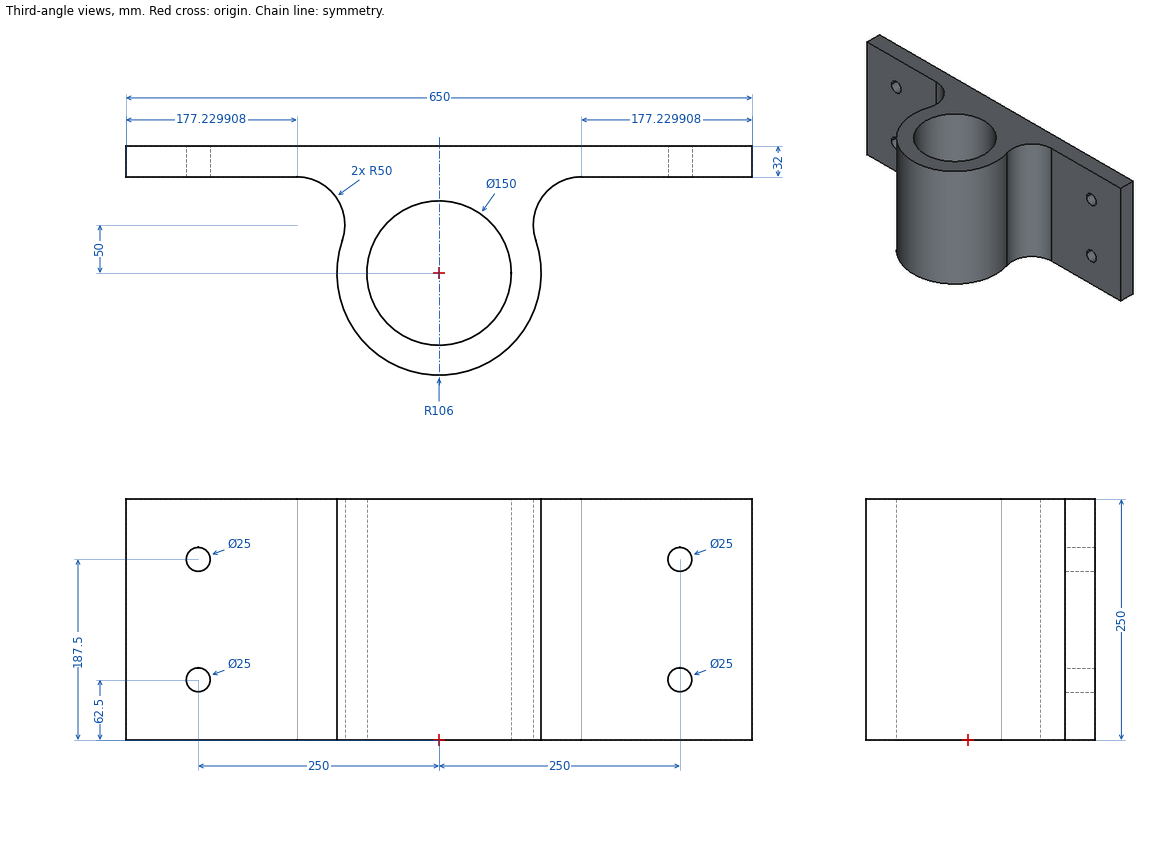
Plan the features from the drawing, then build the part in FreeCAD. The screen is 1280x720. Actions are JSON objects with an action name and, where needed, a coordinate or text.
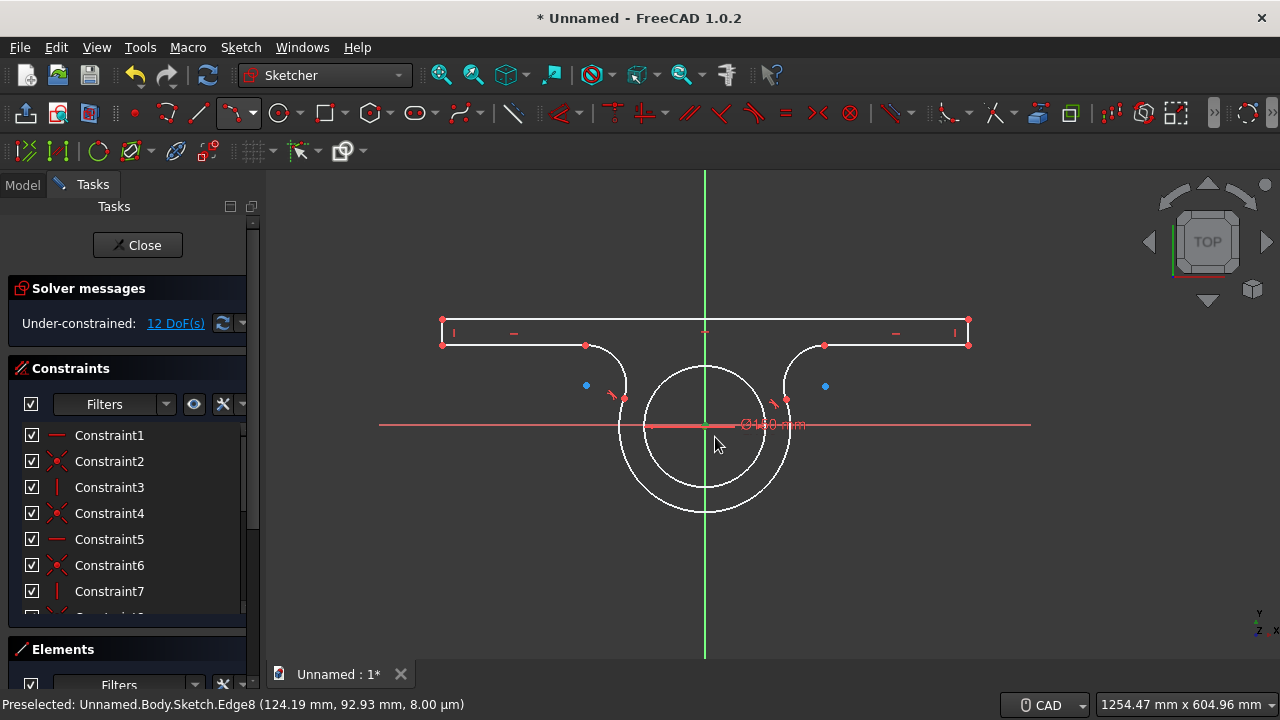
{"action": "key", "text": "c"}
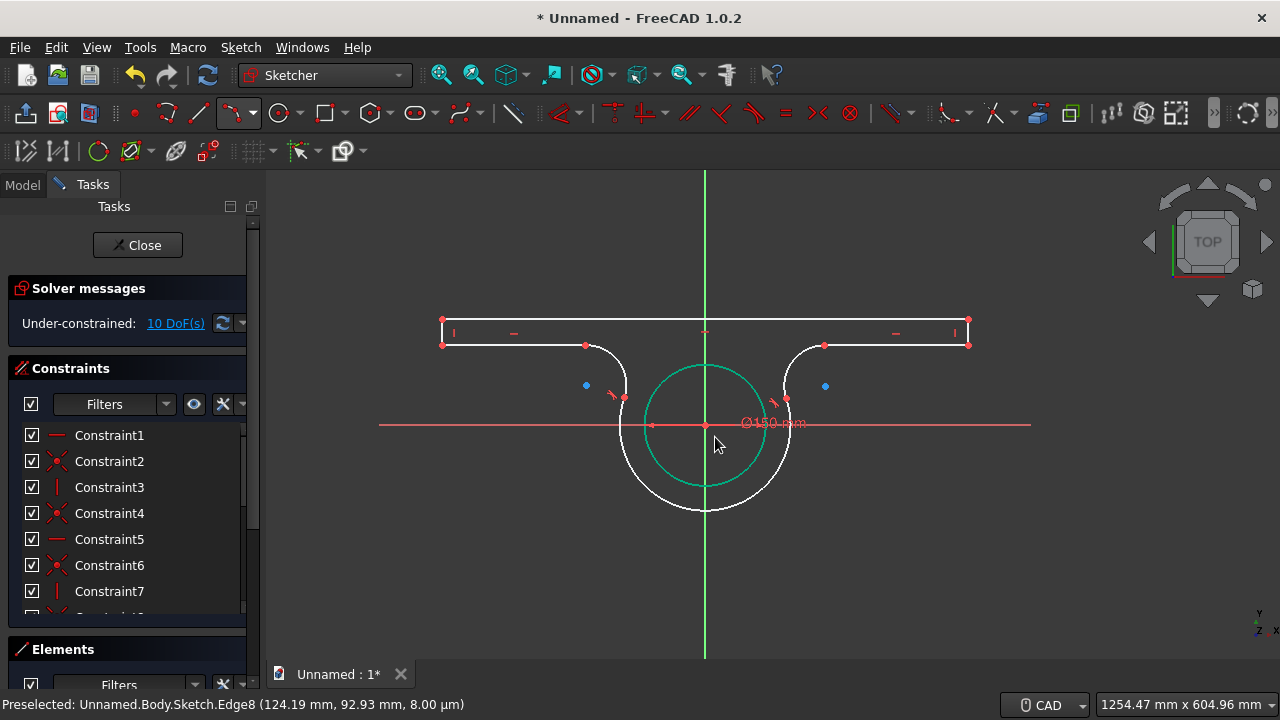
{"action": "left_click", "coordinate": [625, 375]}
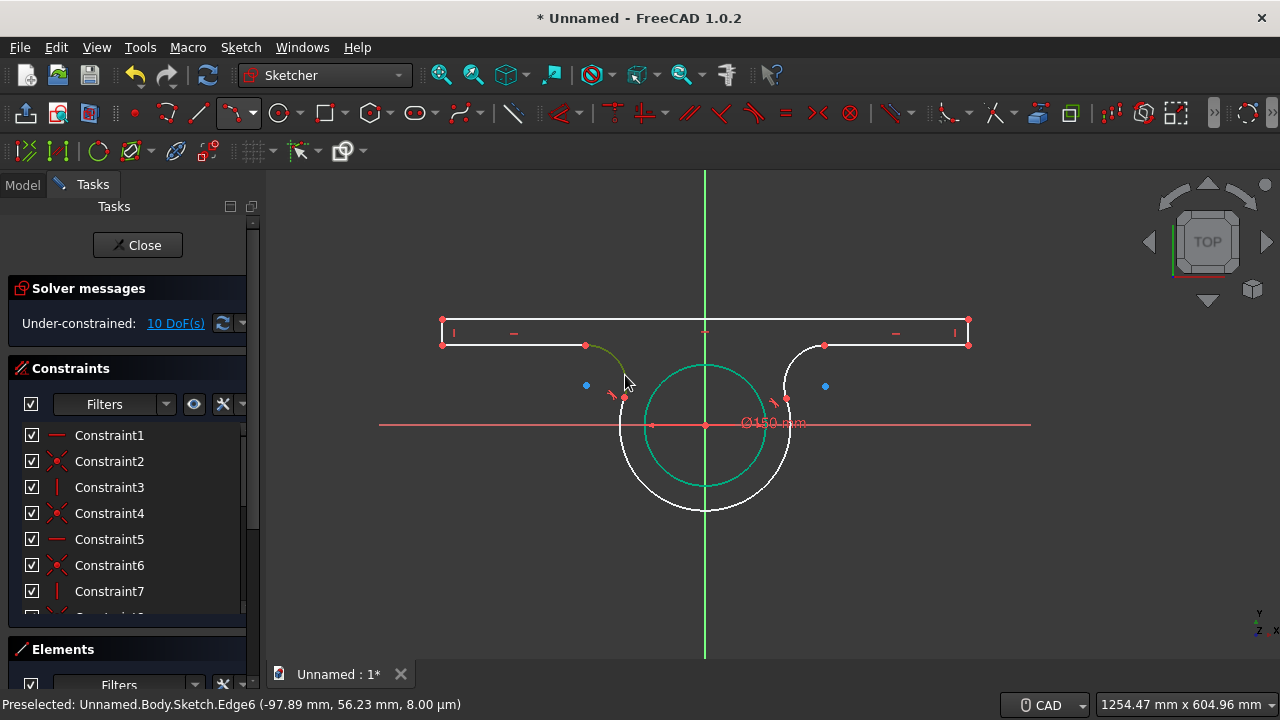
{"action": "left_click", "coordinate": [803, 352]}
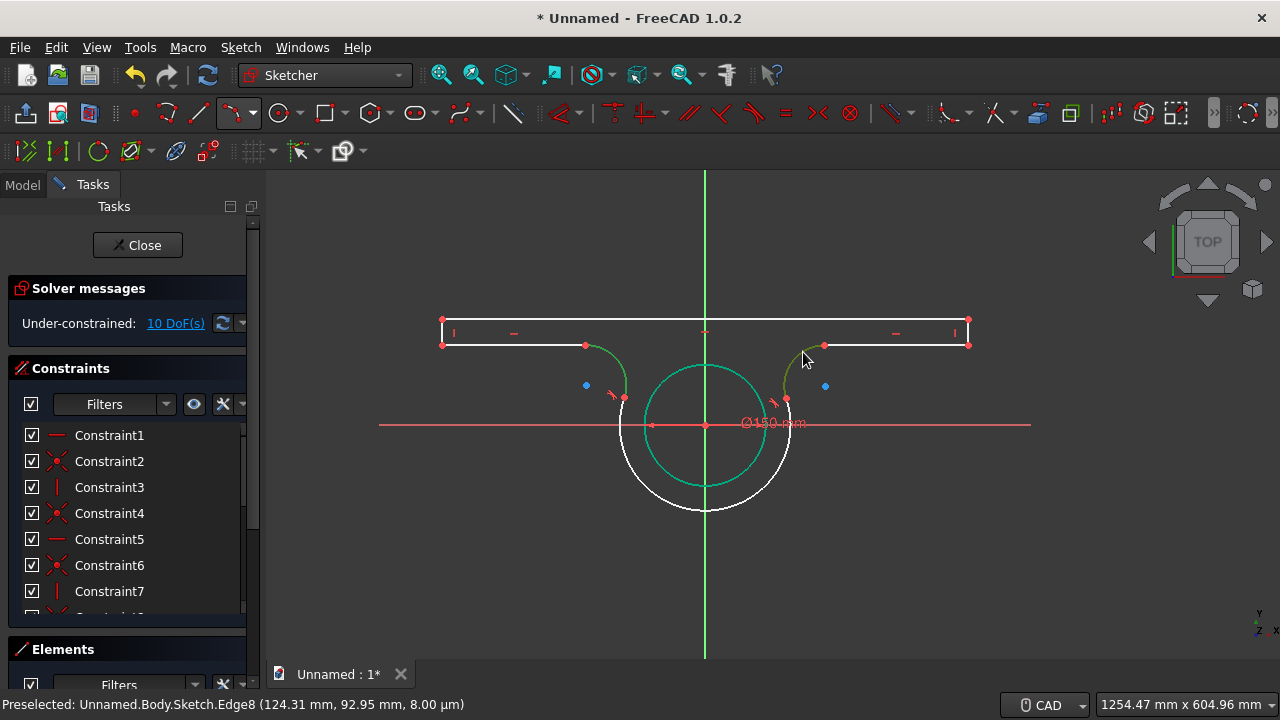
{"action": "left_click", "coordinate": [786, 114]}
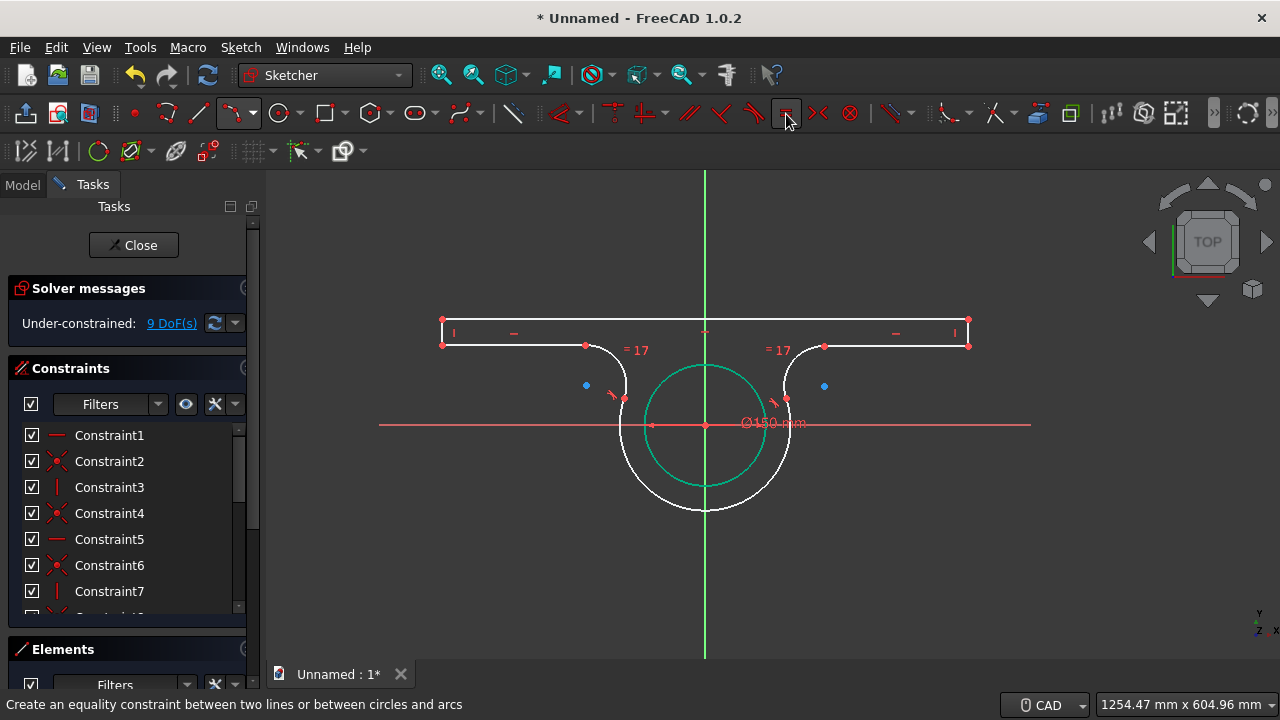
{"action": "left_click", "coordinate": [968, 346]}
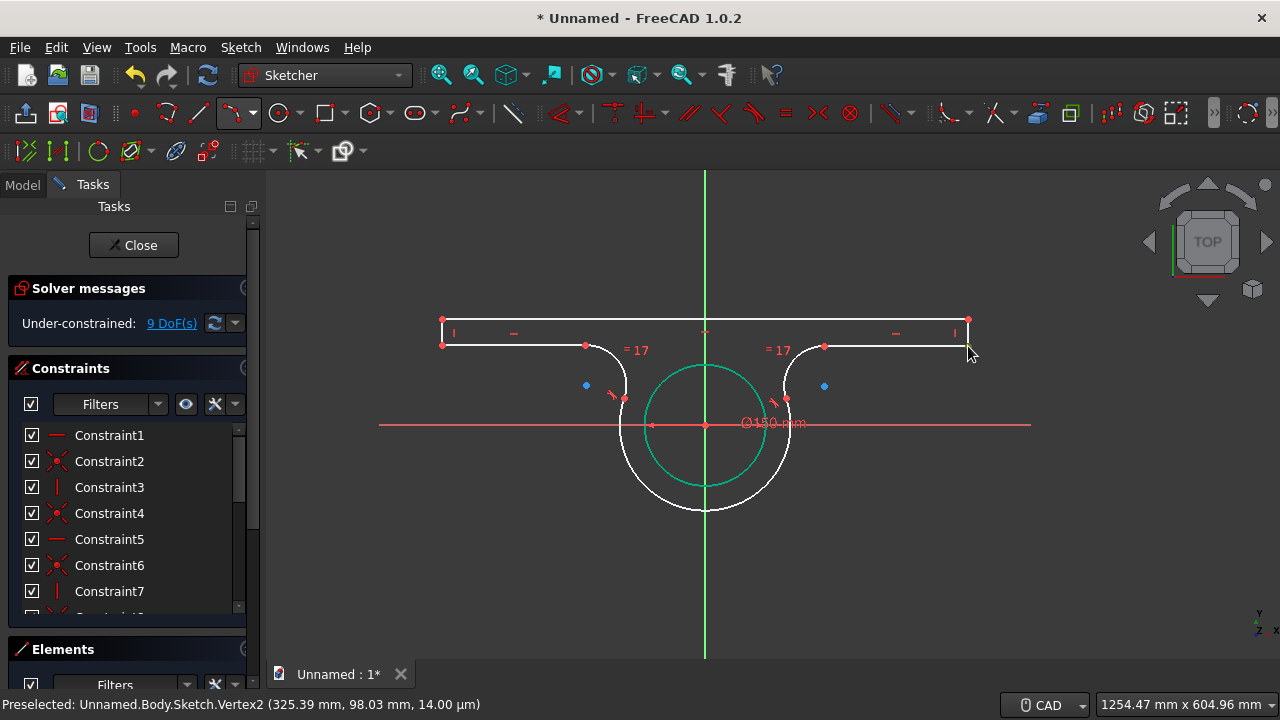
{"action": "left_click", "coordinate": [442, 345]}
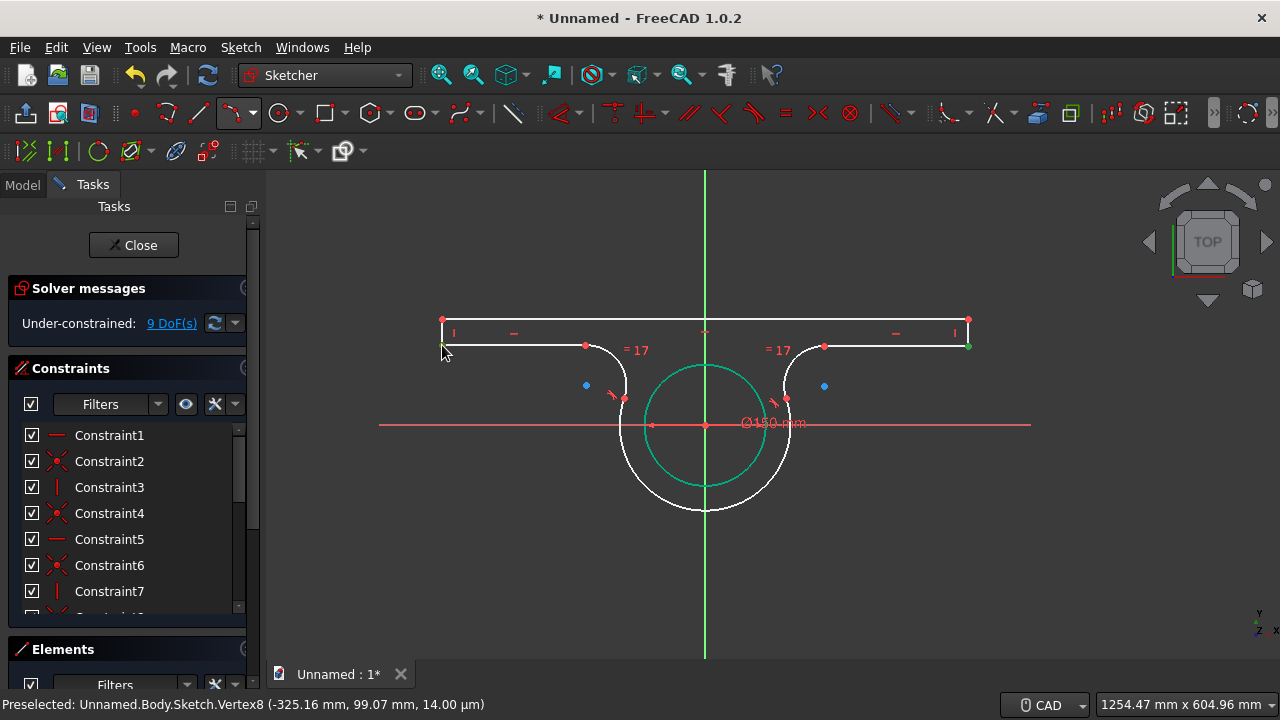
{"action": "left_click", "coordinate": [705, 600]}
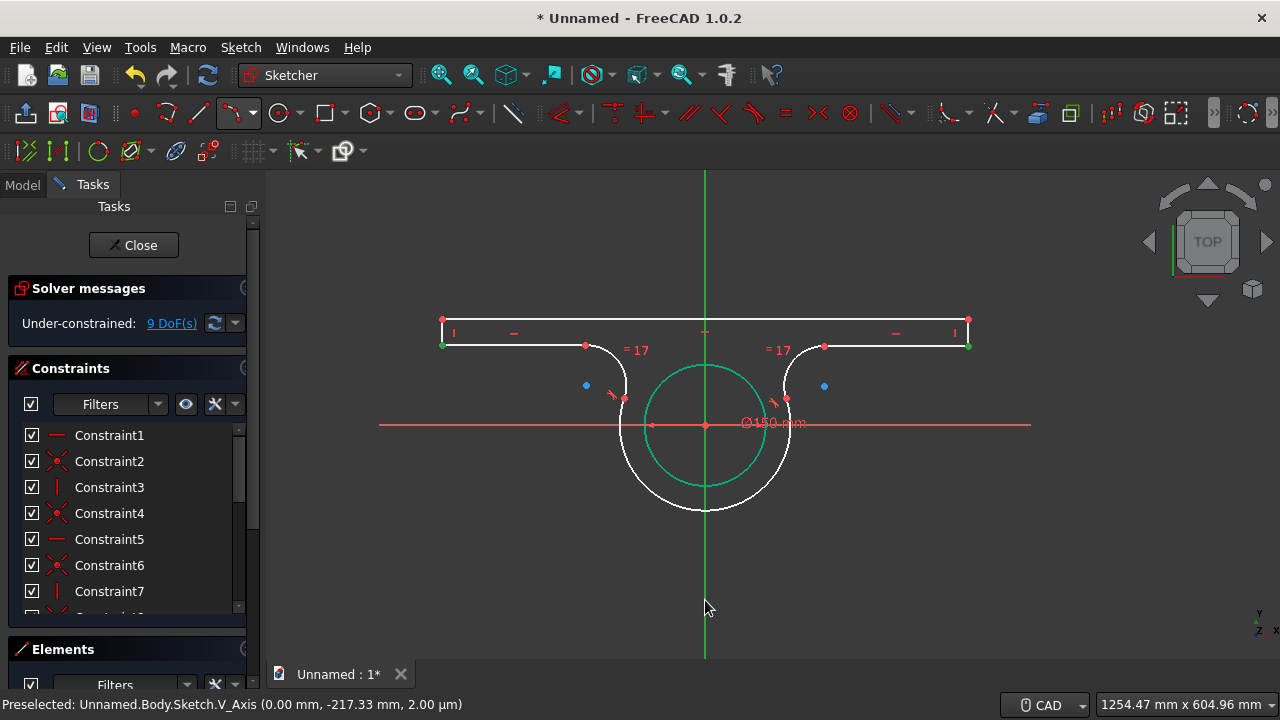
{"action": "left_click", "coordinate": [818, 114]}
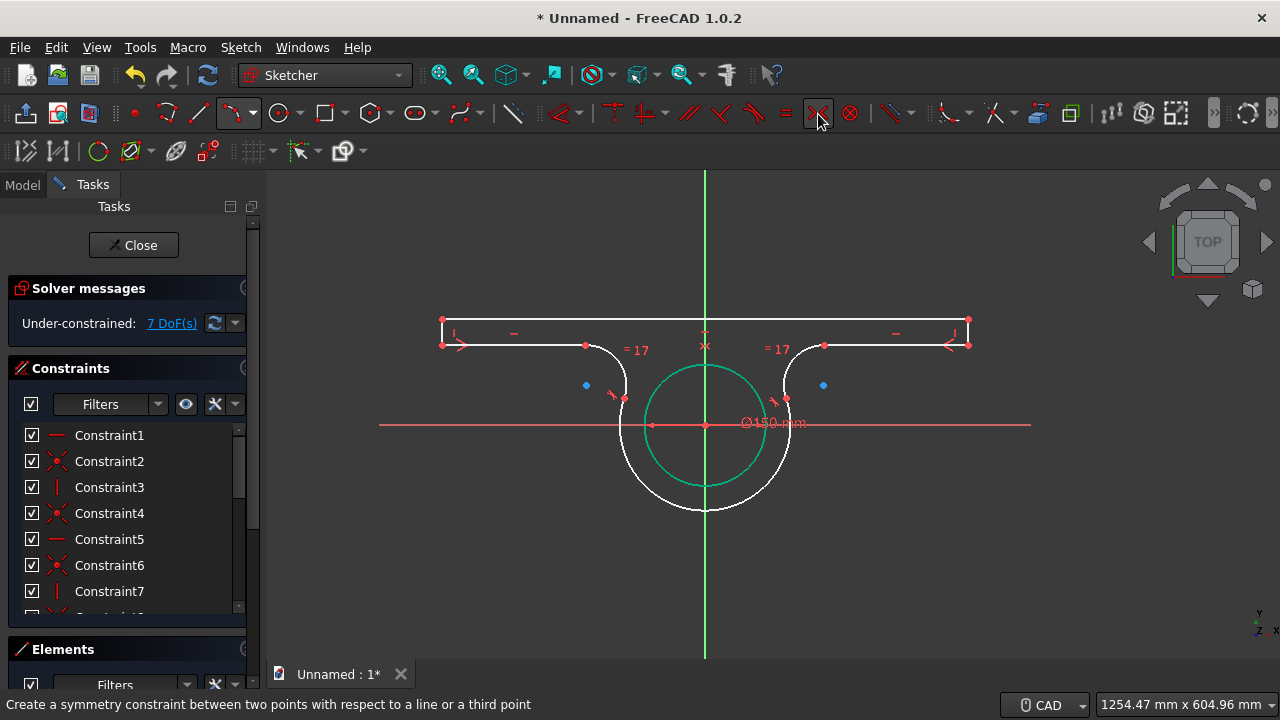
{"action": "left_click", "coordinate": [560, 114]}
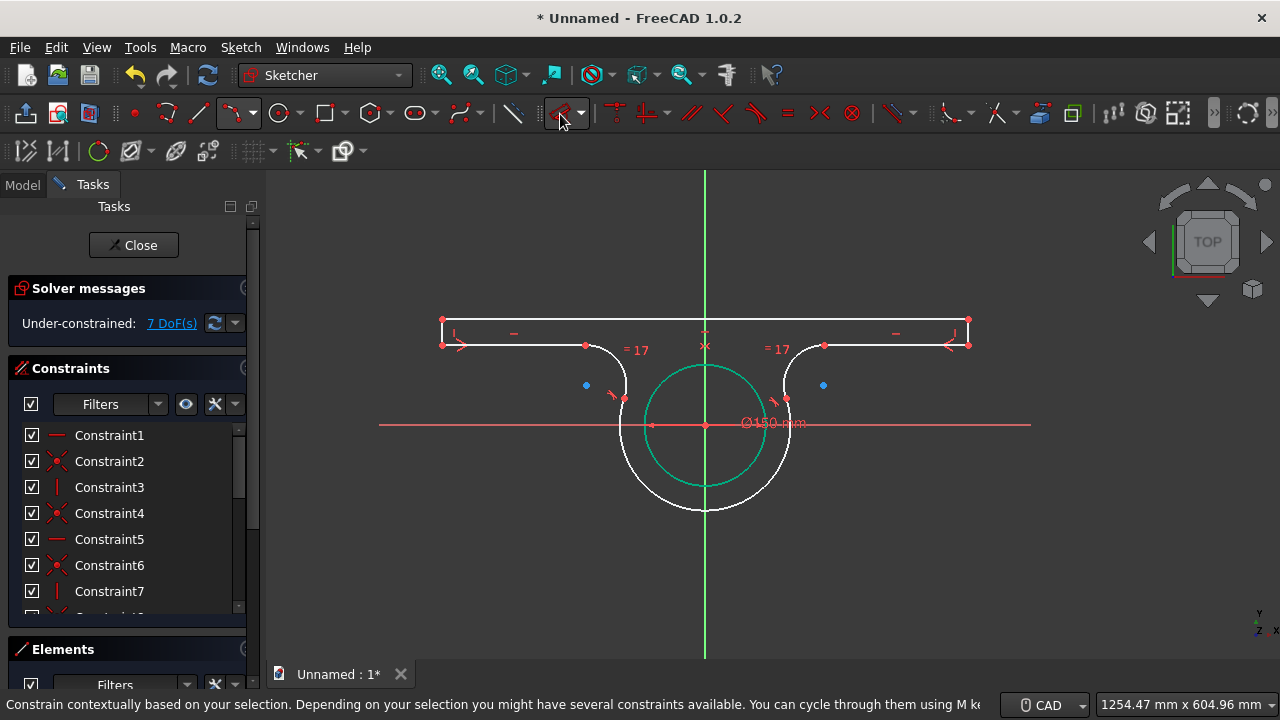
{"action": "left_click", "coordinate": [625, 375]}
{"action": "left_click", "coordinate": [656, 367]}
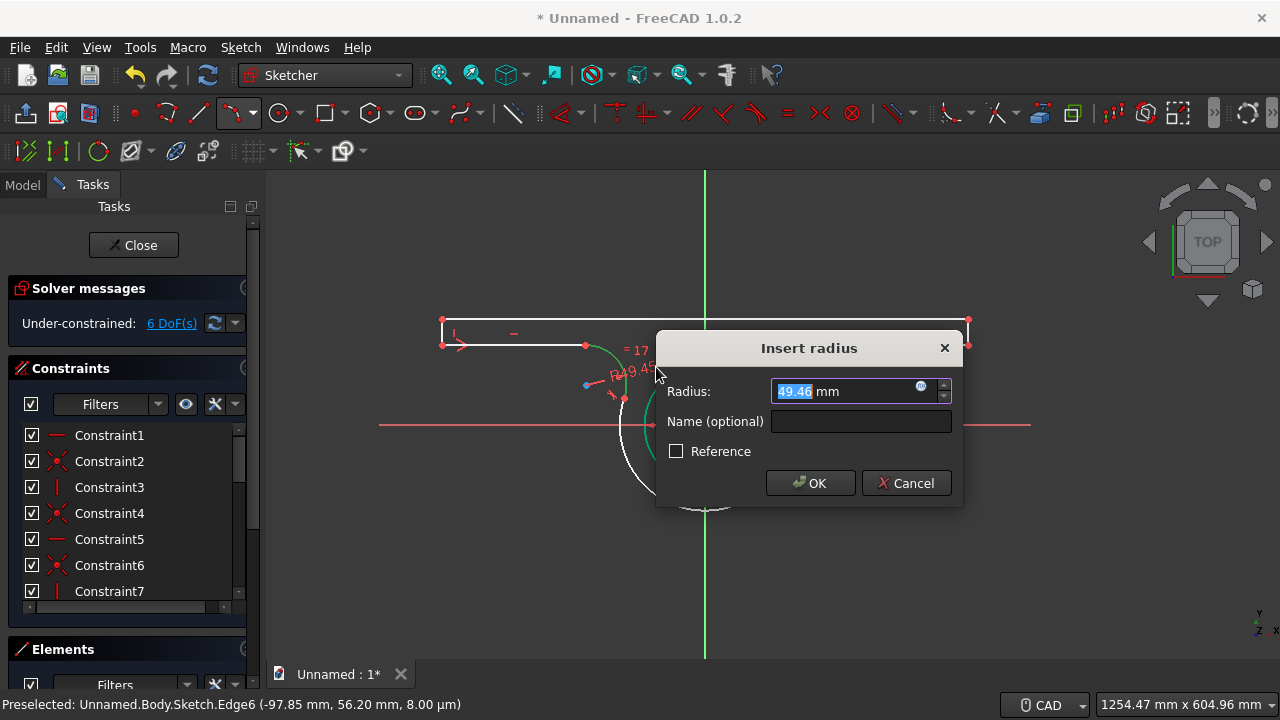
{"action": "type", "text": "50"}
{"action": "key", "text": "Return"}